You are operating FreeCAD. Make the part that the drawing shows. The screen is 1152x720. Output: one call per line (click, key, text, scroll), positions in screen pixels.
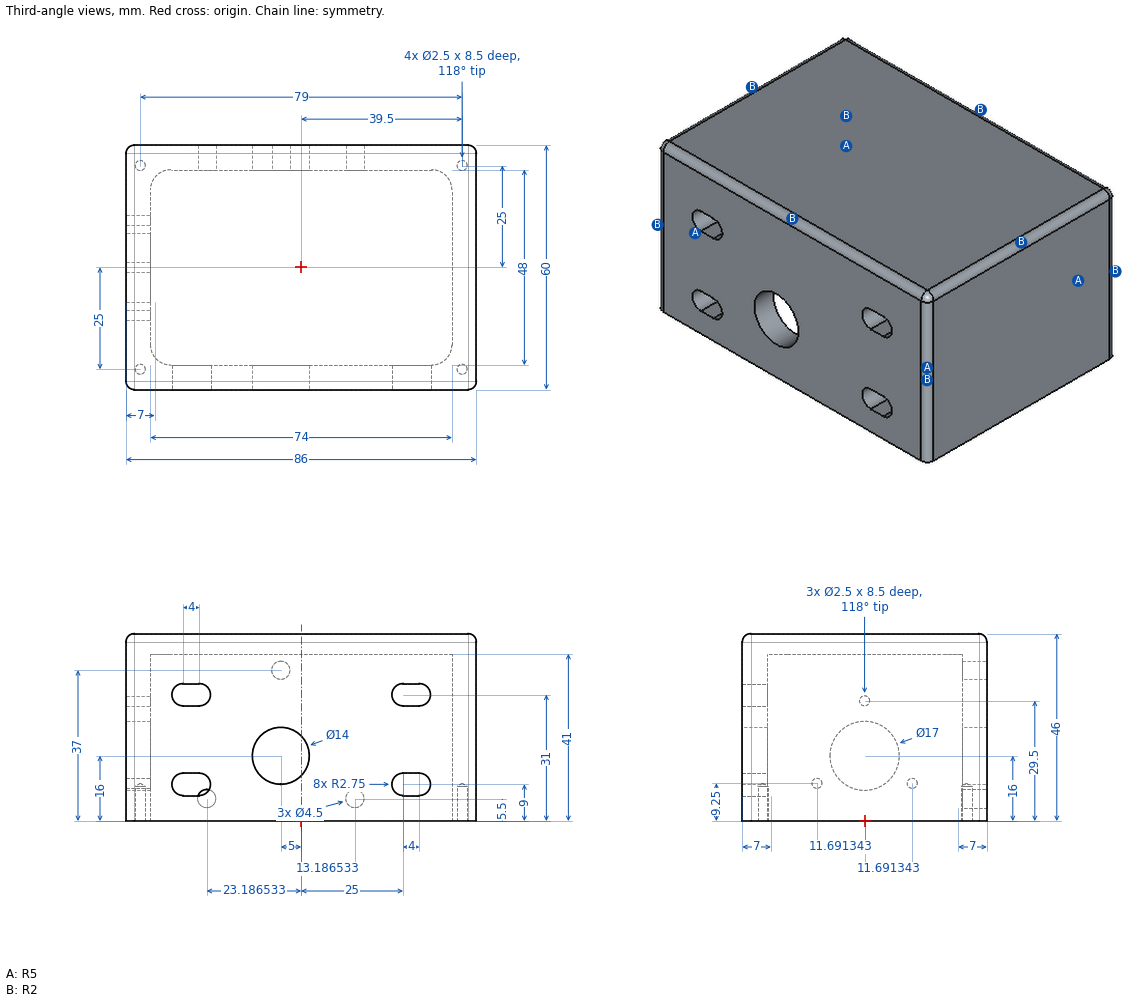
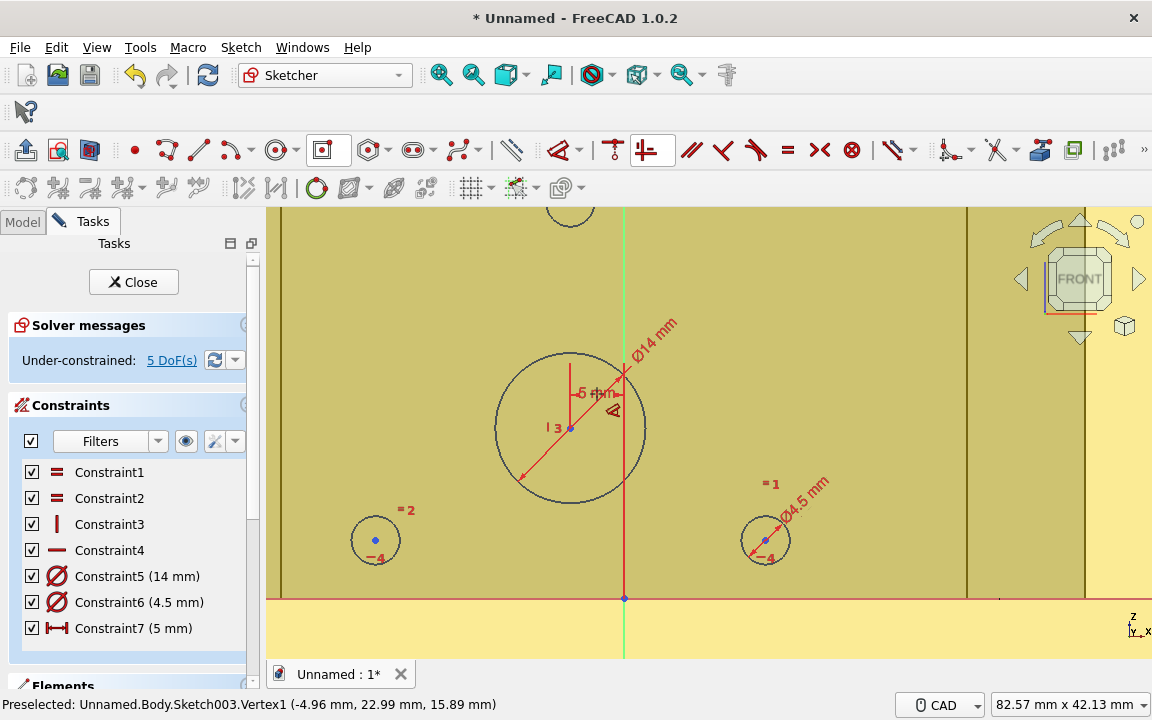
click(570, 428)
click(658, 513)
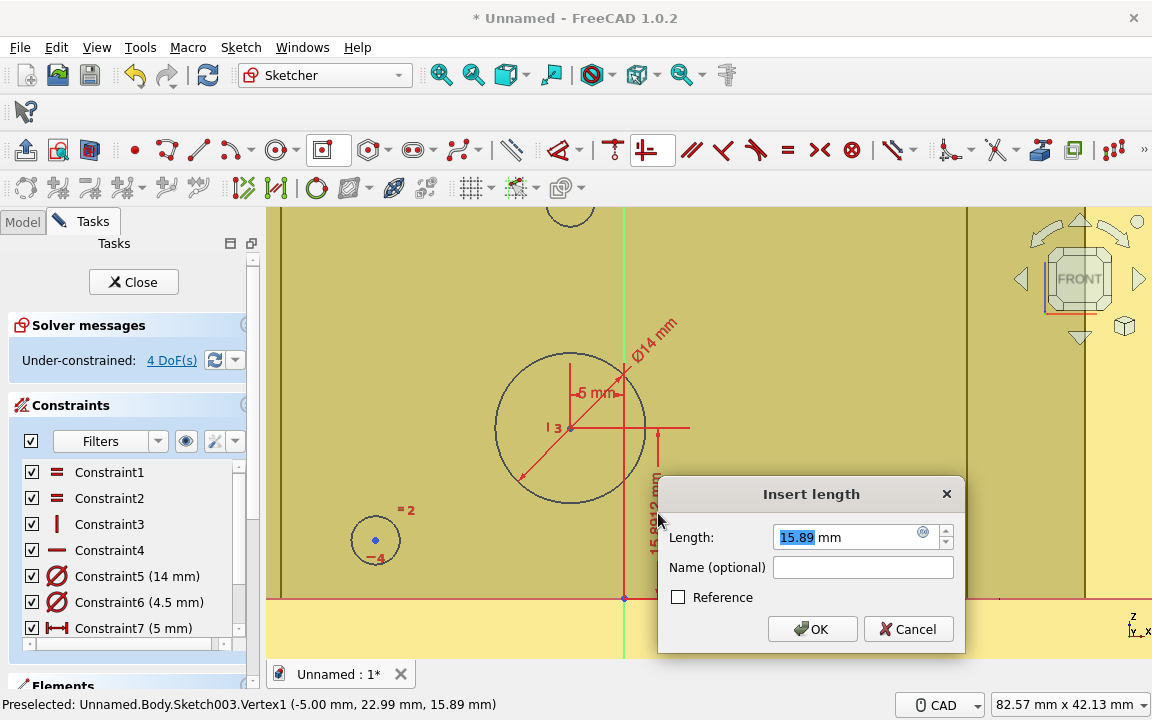
text(16)
key(Return)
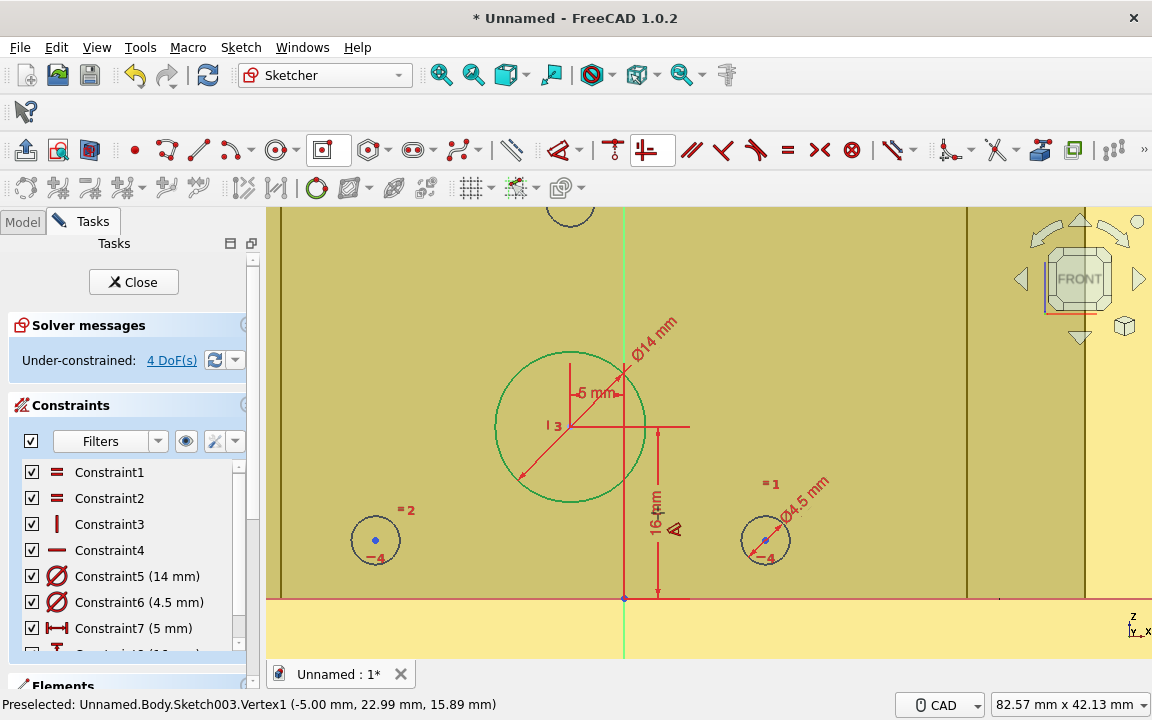
scroll(783, 524, down, 2)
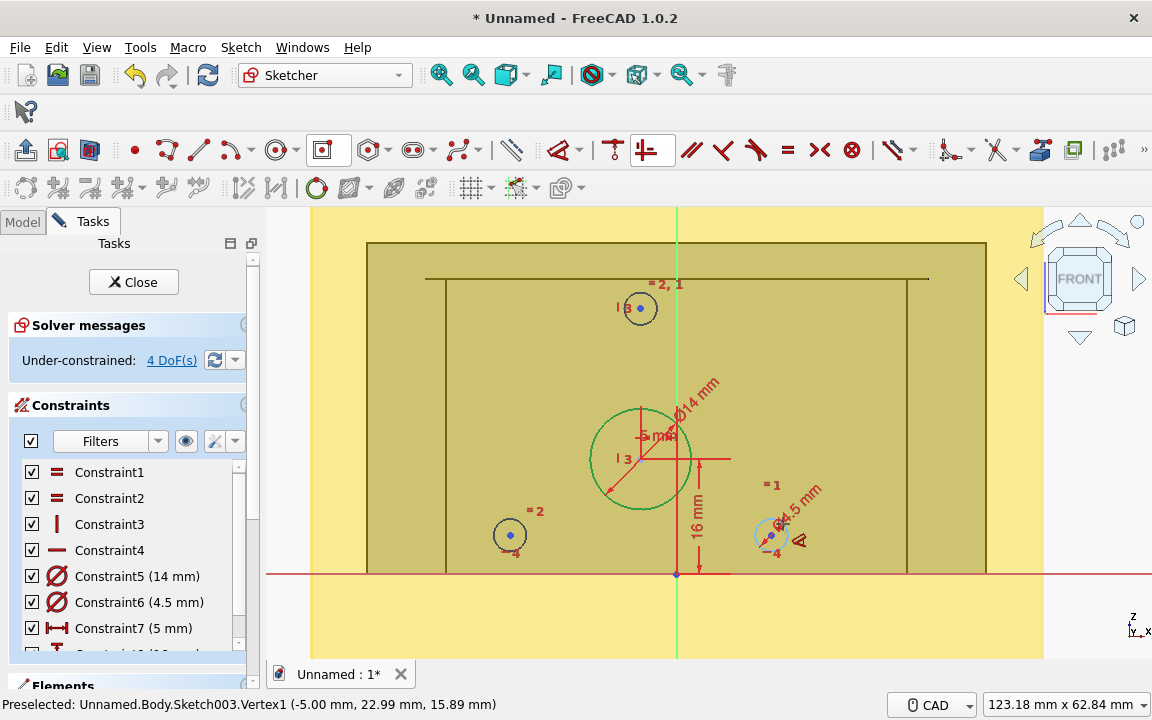
click(641, 309)
click(711, 380)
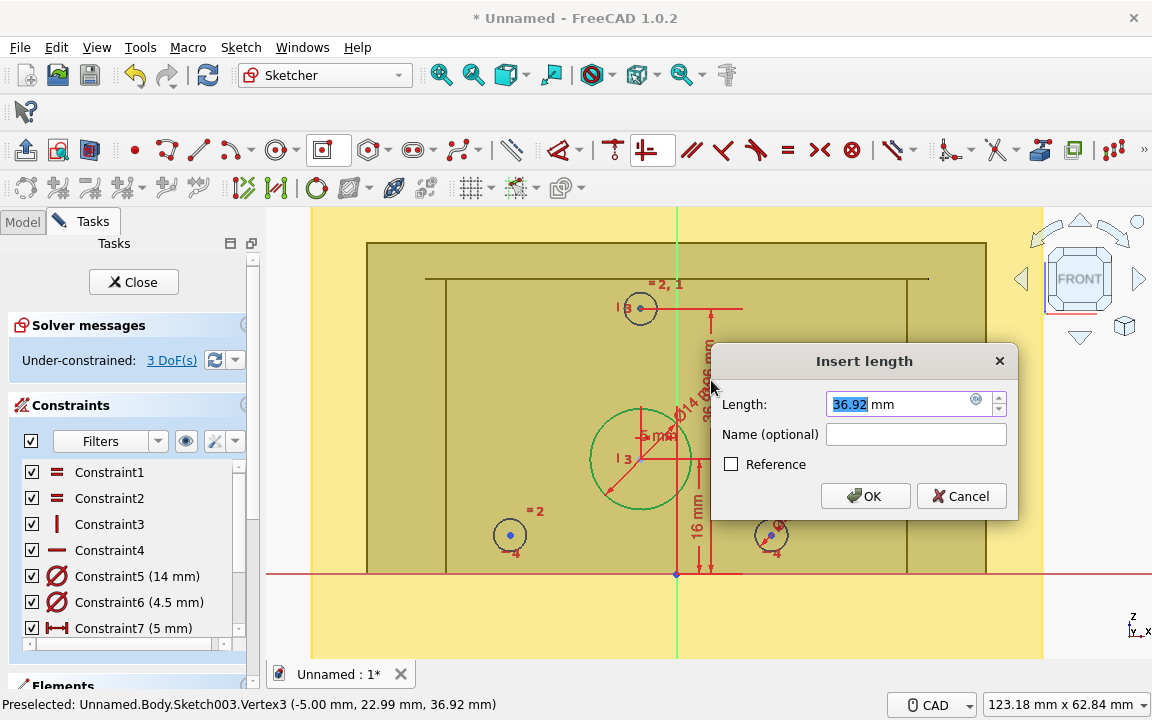
text(37)
key(Return)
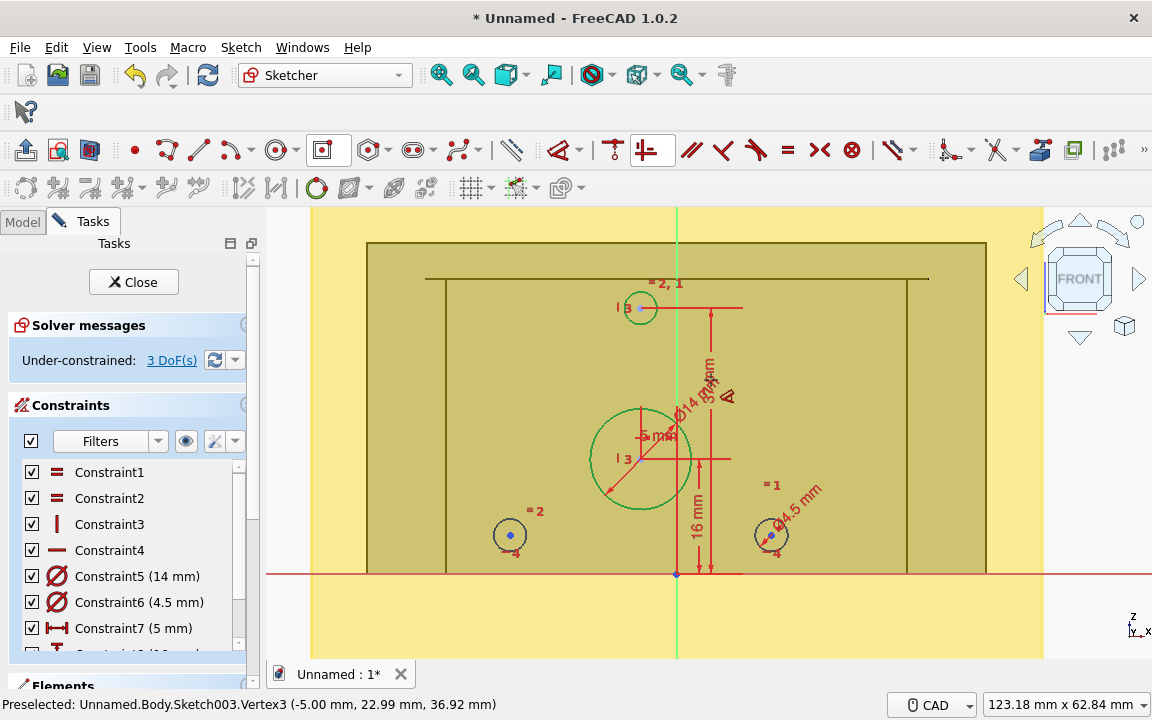
click(772, 535)
click(806, 555)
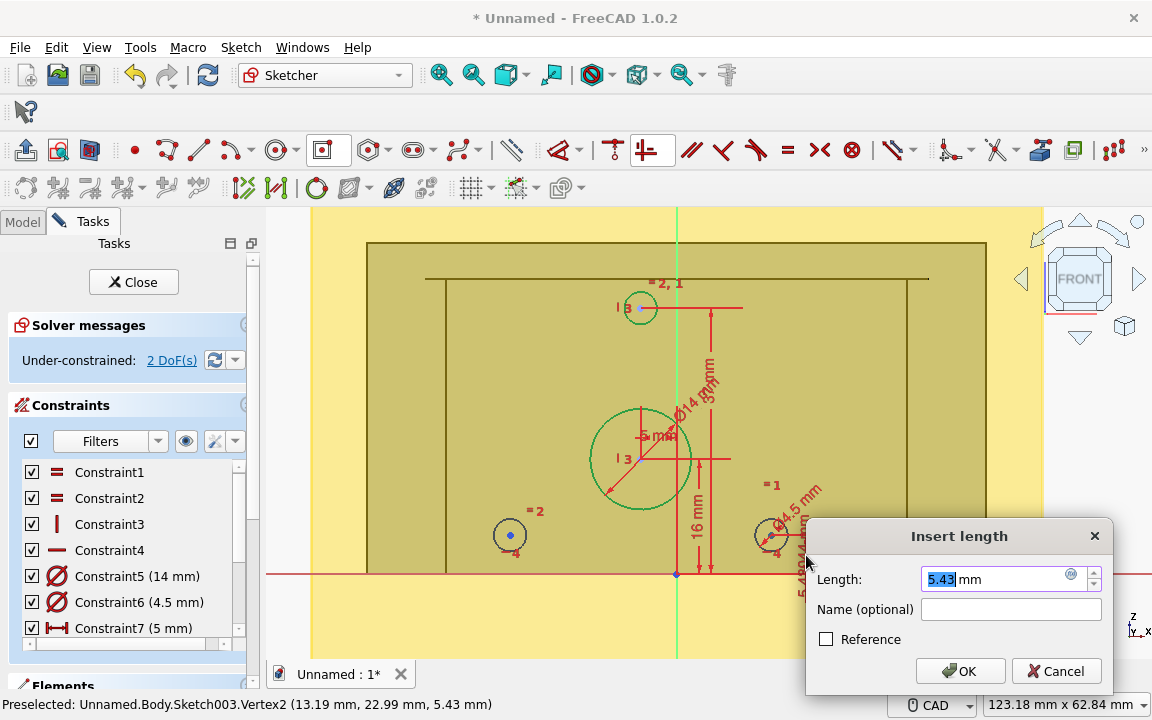
text(5.5)
key(Return)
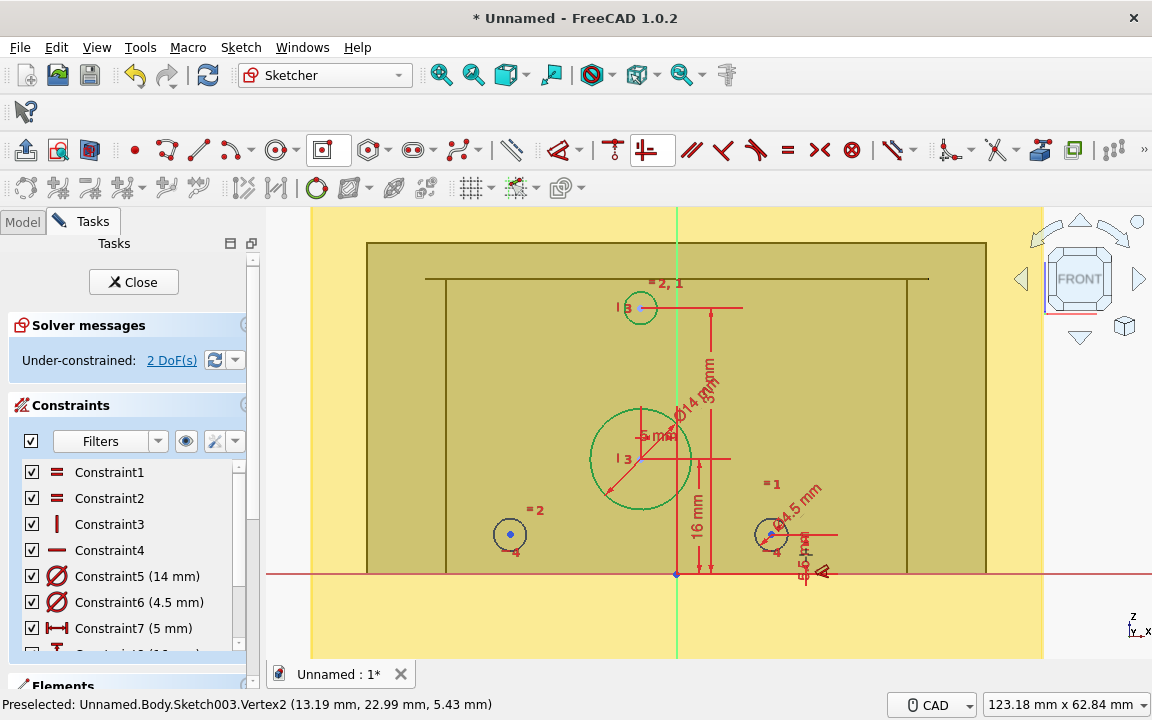
click(772, 535)
click(724, 608)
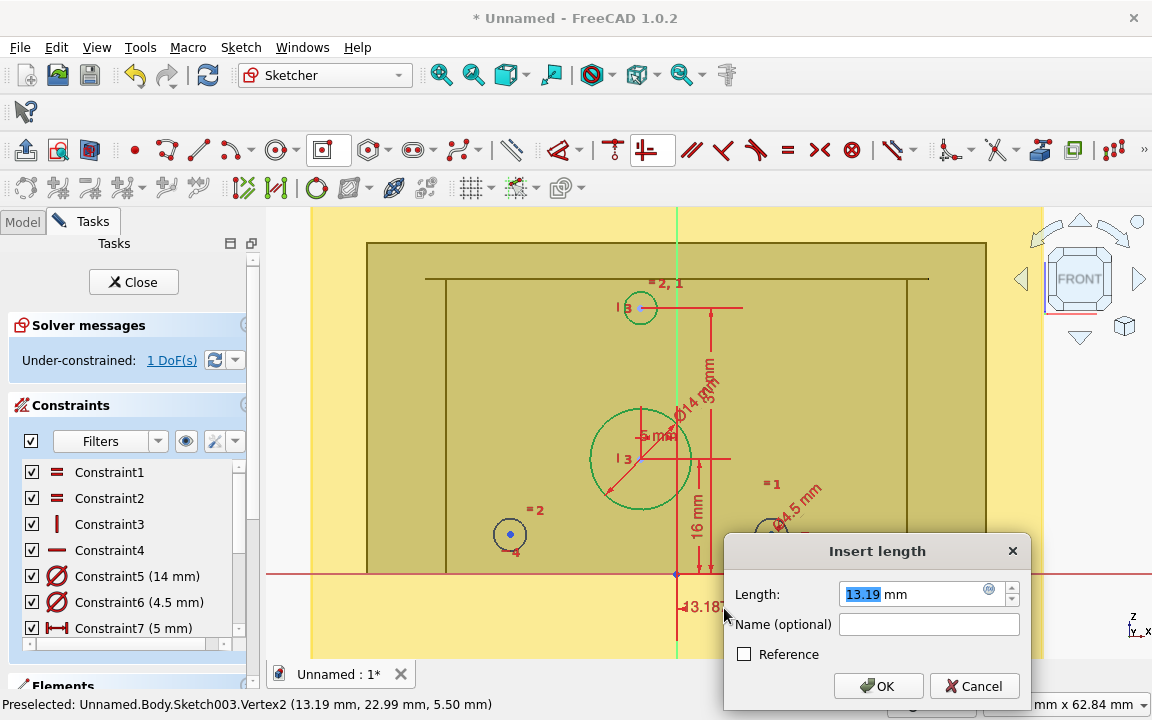
text(13.186533)
key(Return)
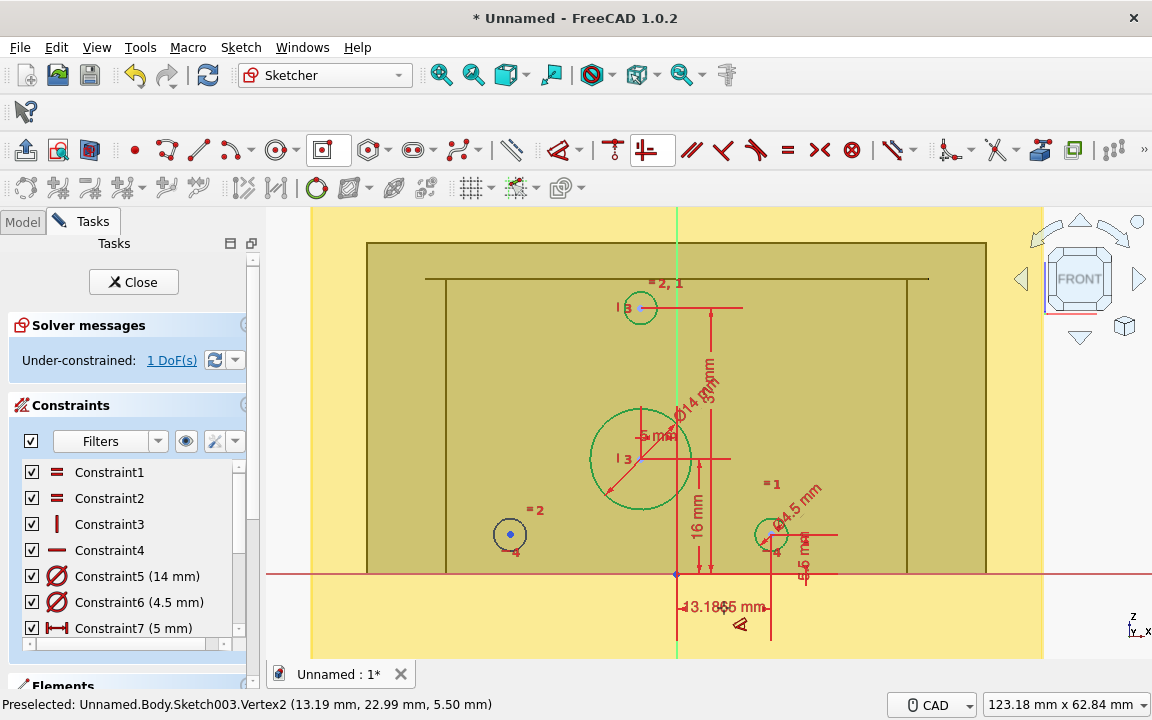
click(510, 535)
click(593, 608)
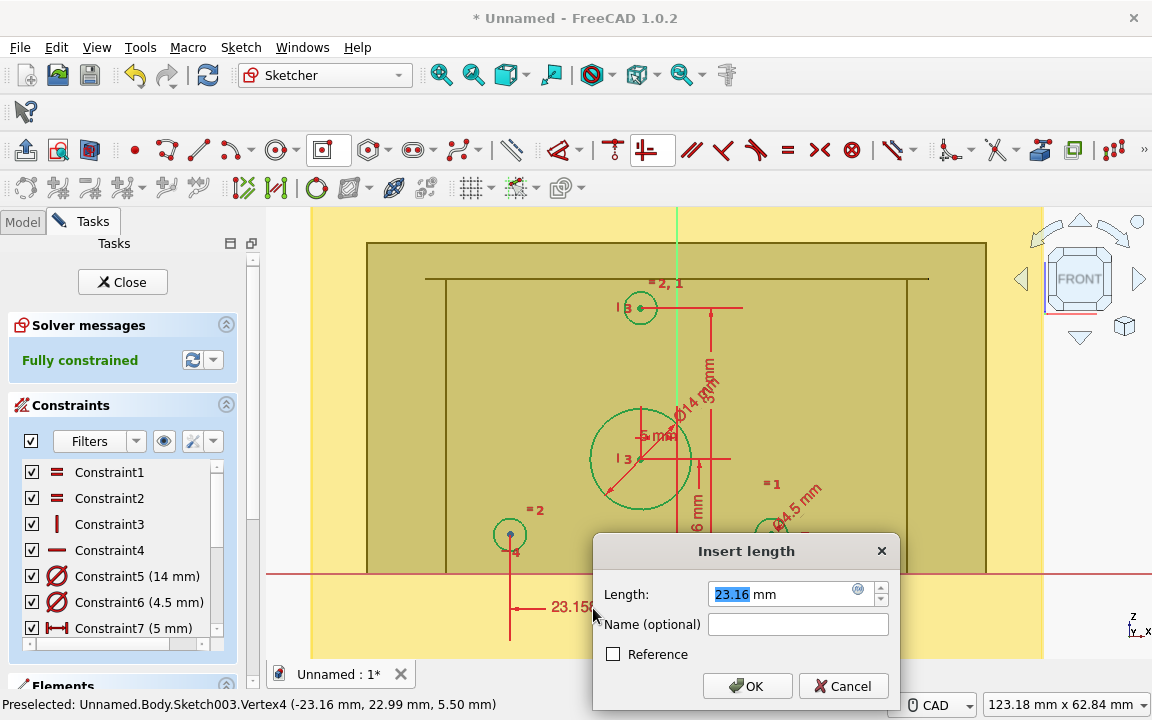
text(23.186533)
key(Return)
key(Escape)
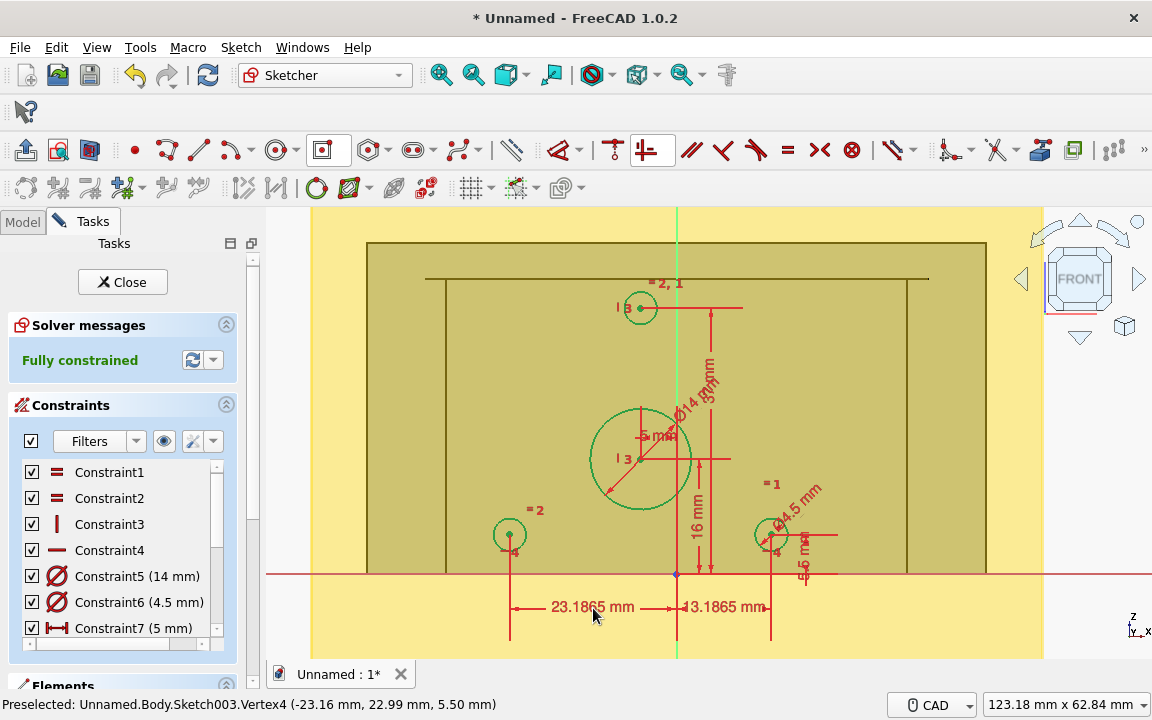
click(123, 282)